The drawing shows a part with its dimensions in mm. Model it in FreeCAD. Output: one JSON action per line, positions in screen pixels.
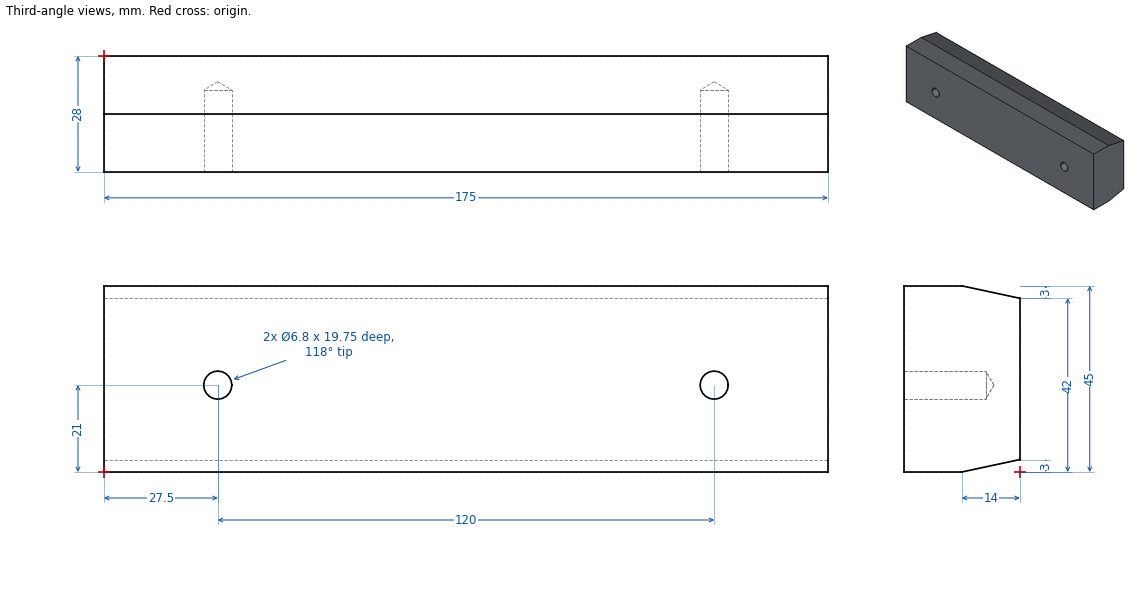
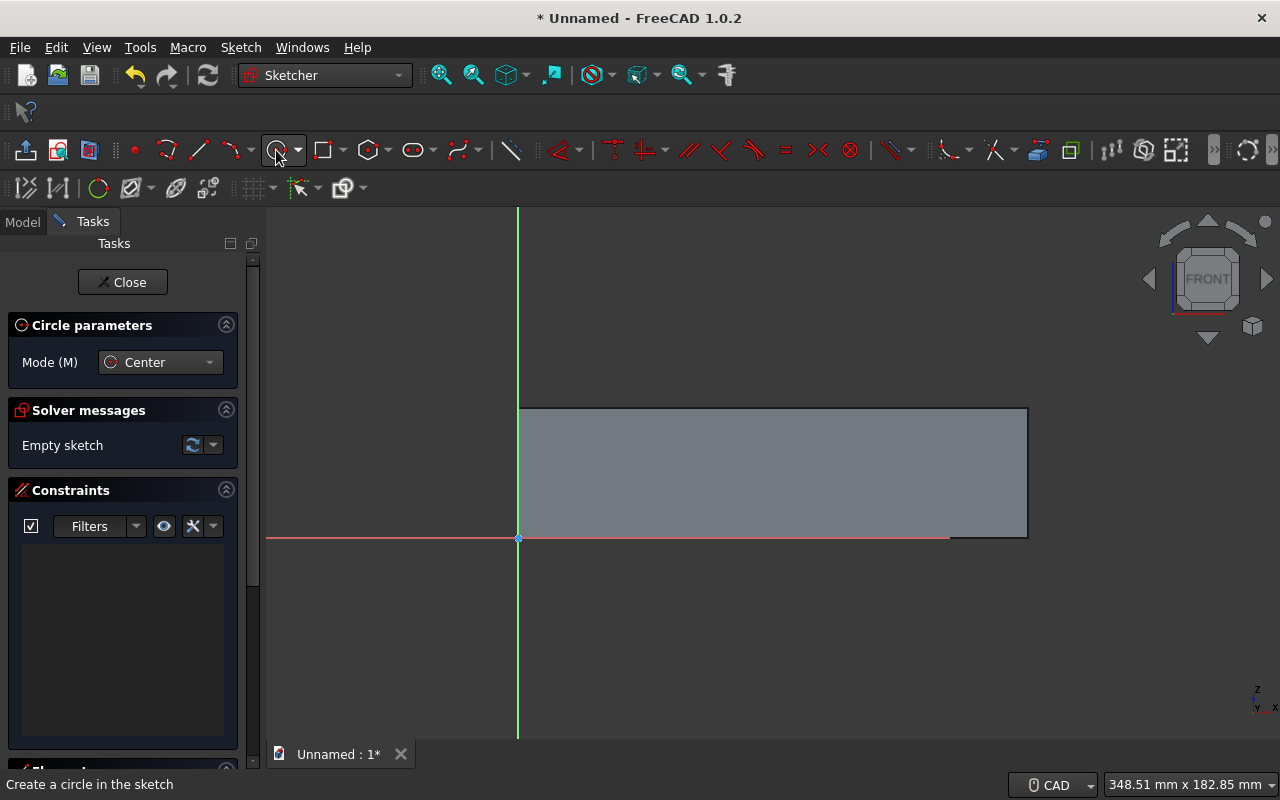
{"action": "scroll", "coordinate": [598, 477], "scroll_direction": "up", "scroll_amount": 5}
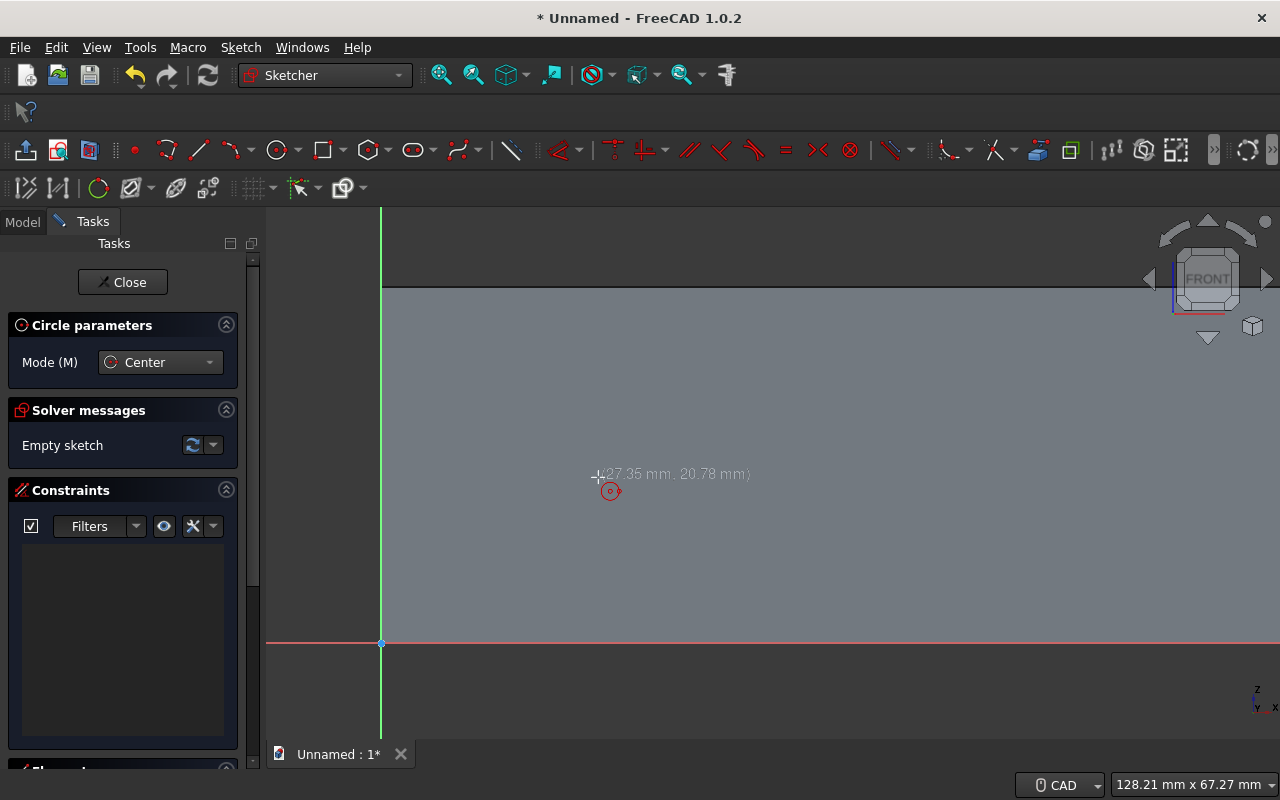
{"action": "left_click", "coordinate": [599, 477]}
{"action": "left_click", "coordinate": [618, 458]}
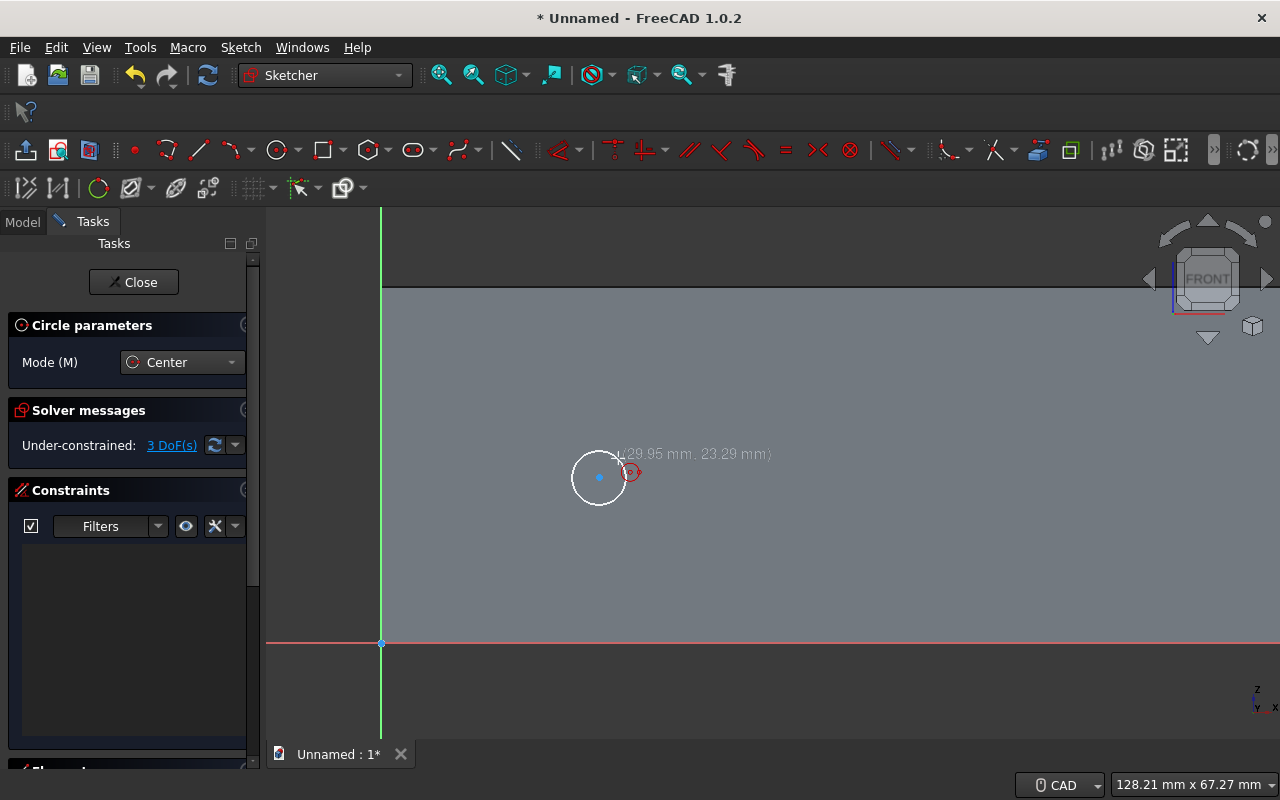
{"action": "scroll", "coordinate": [481, 413], "scroll_direction": "down", "scroll_amount": 4}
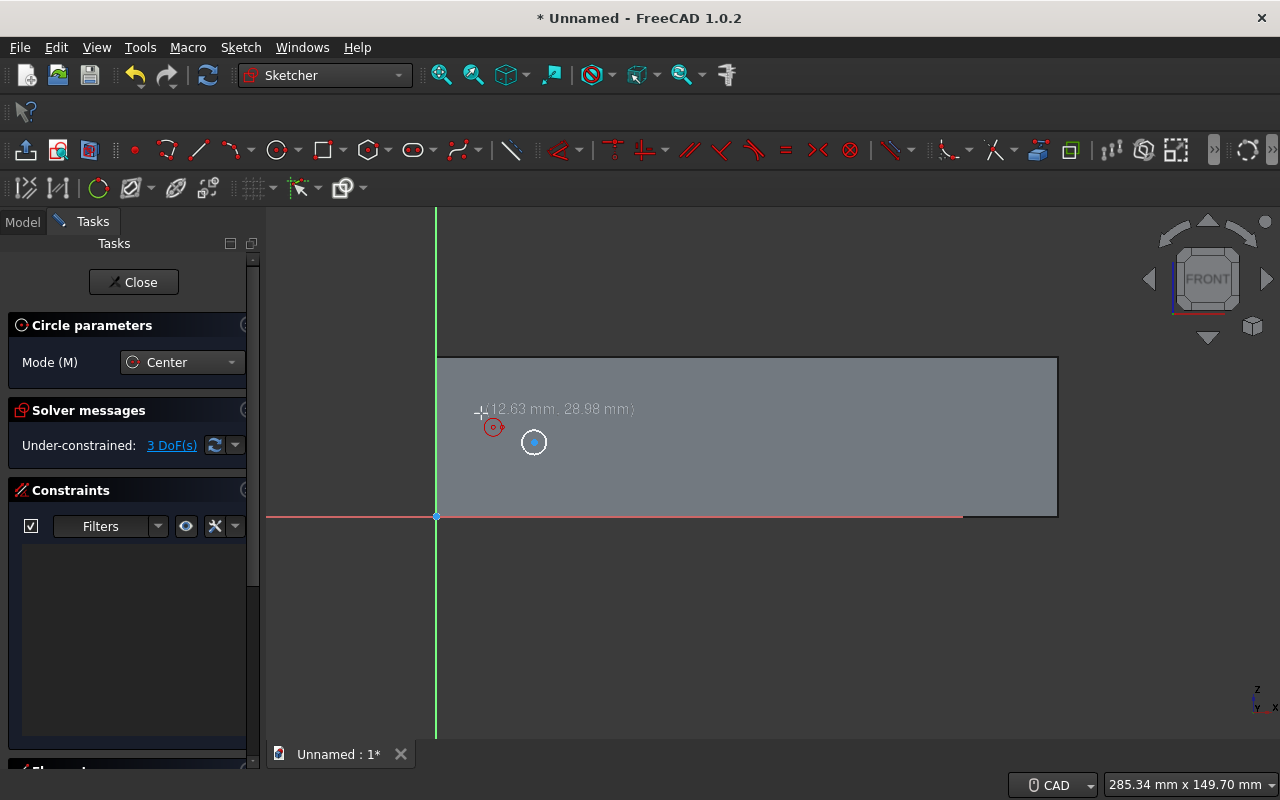
{"action": "scroll", "coordinate": [960, 442], "scroll_direction": "up", "scroll_amount": 4}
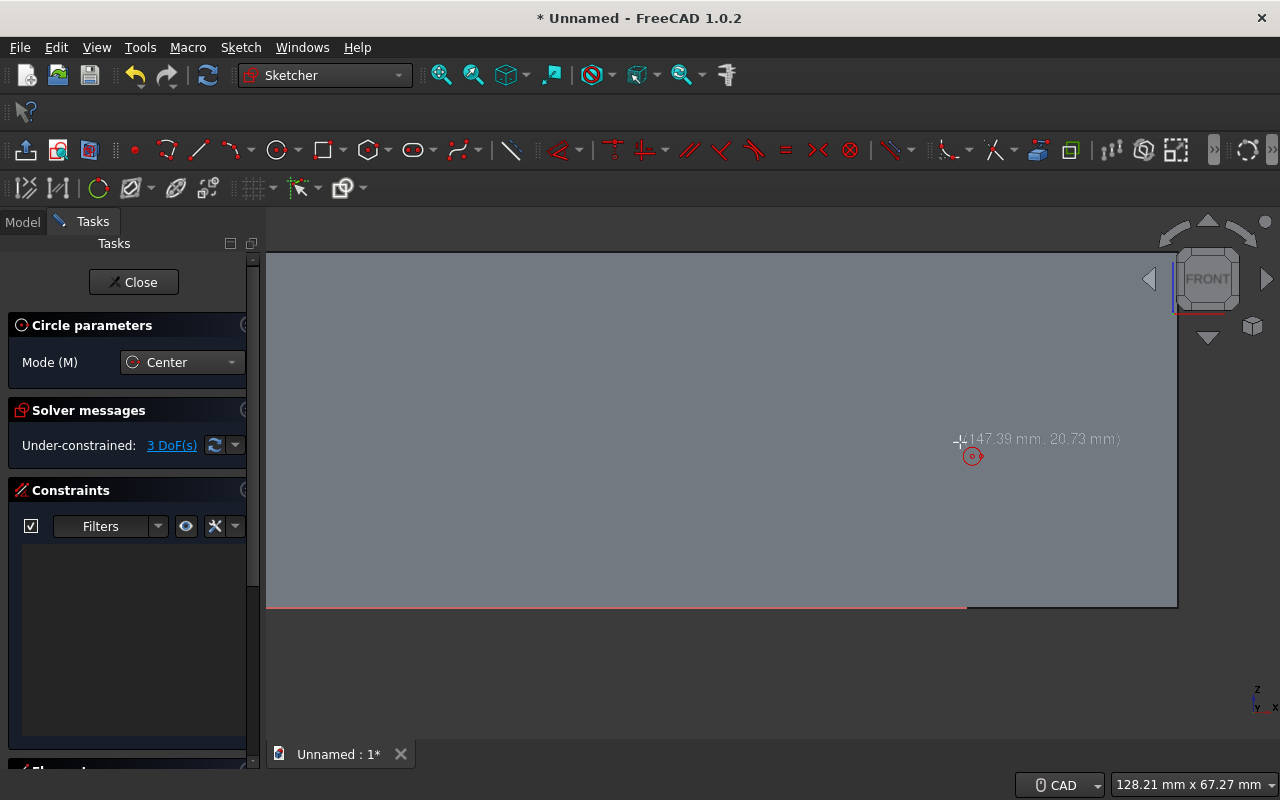
{"action": "left_click", "coordinate": [960, 442]}
{"action": "left_click", "coordinate": [979, 422]}
{"action": "key", "text": "Escape"}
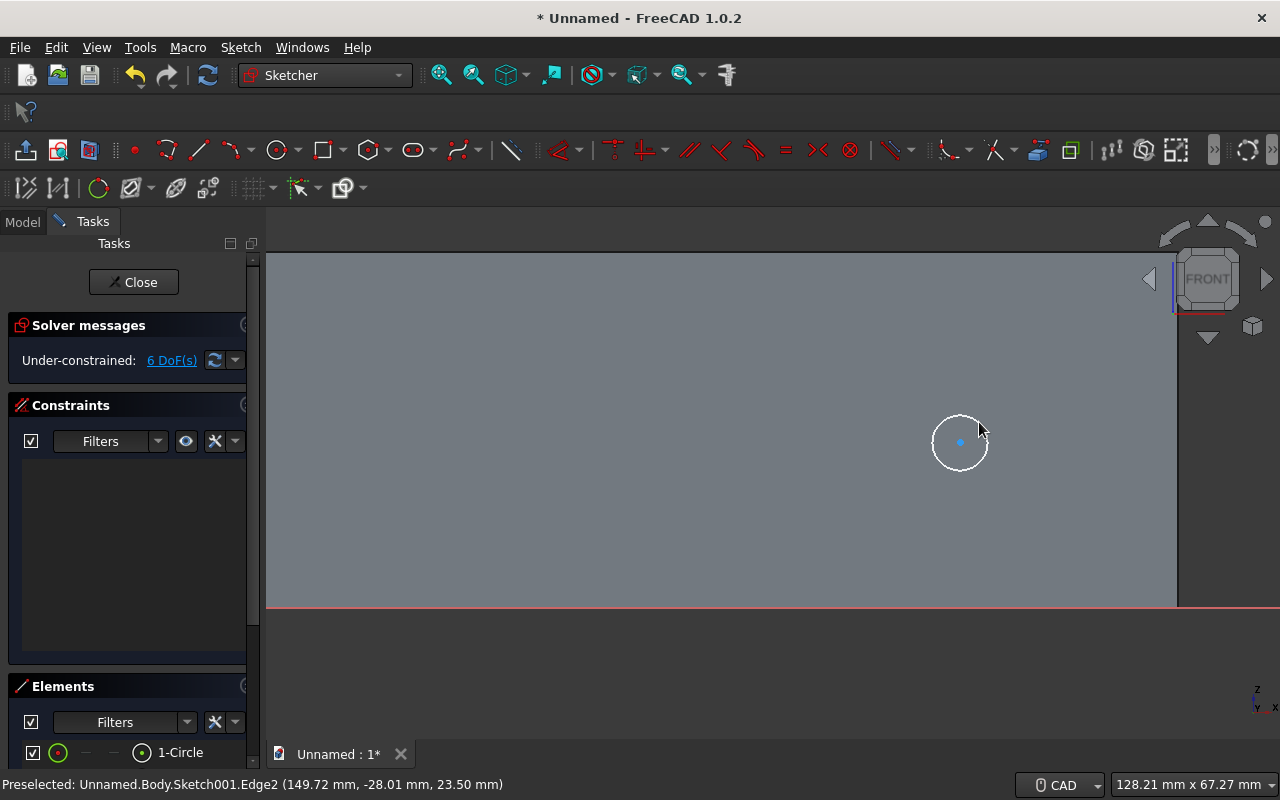
{"action": "scroll", "coordinate": [961, 442], "scroll_direction": "down", "scroll_amount": 4}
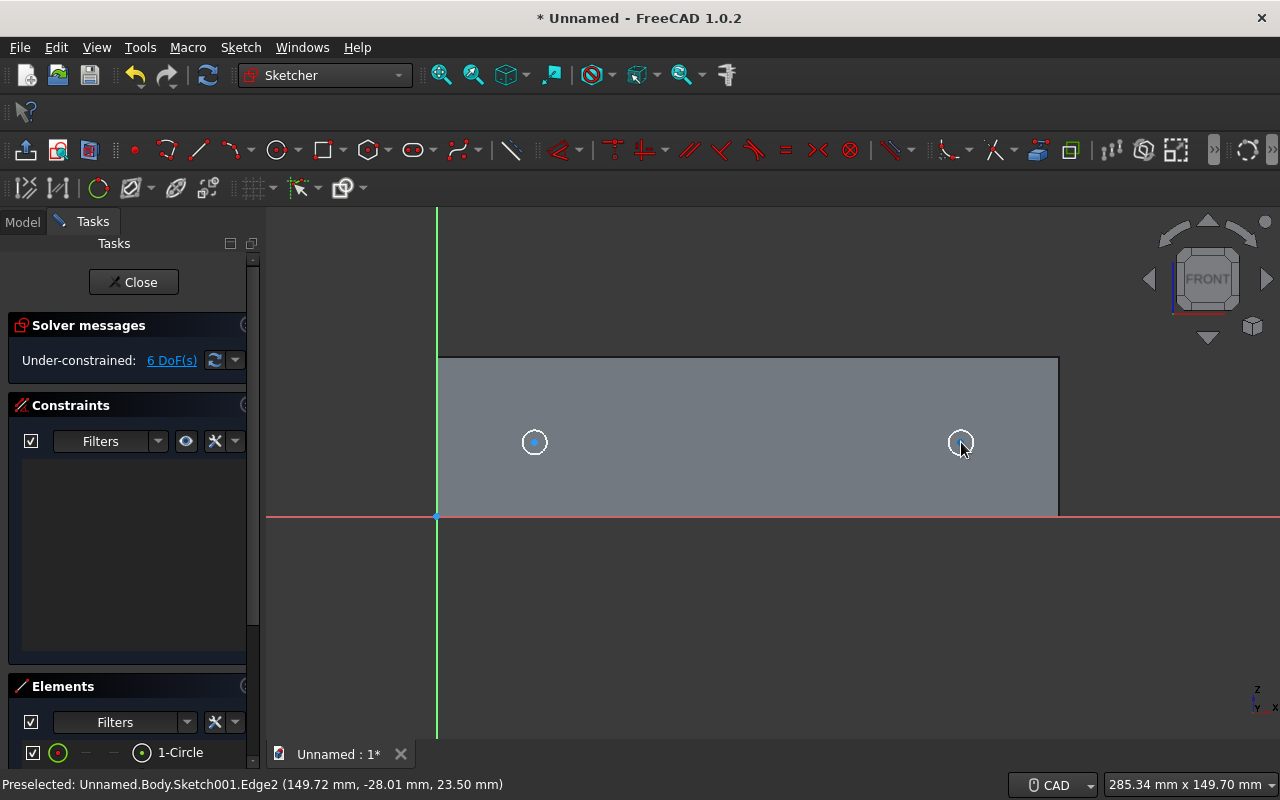
{"action": "left_click", "coordinate": [543, 434]}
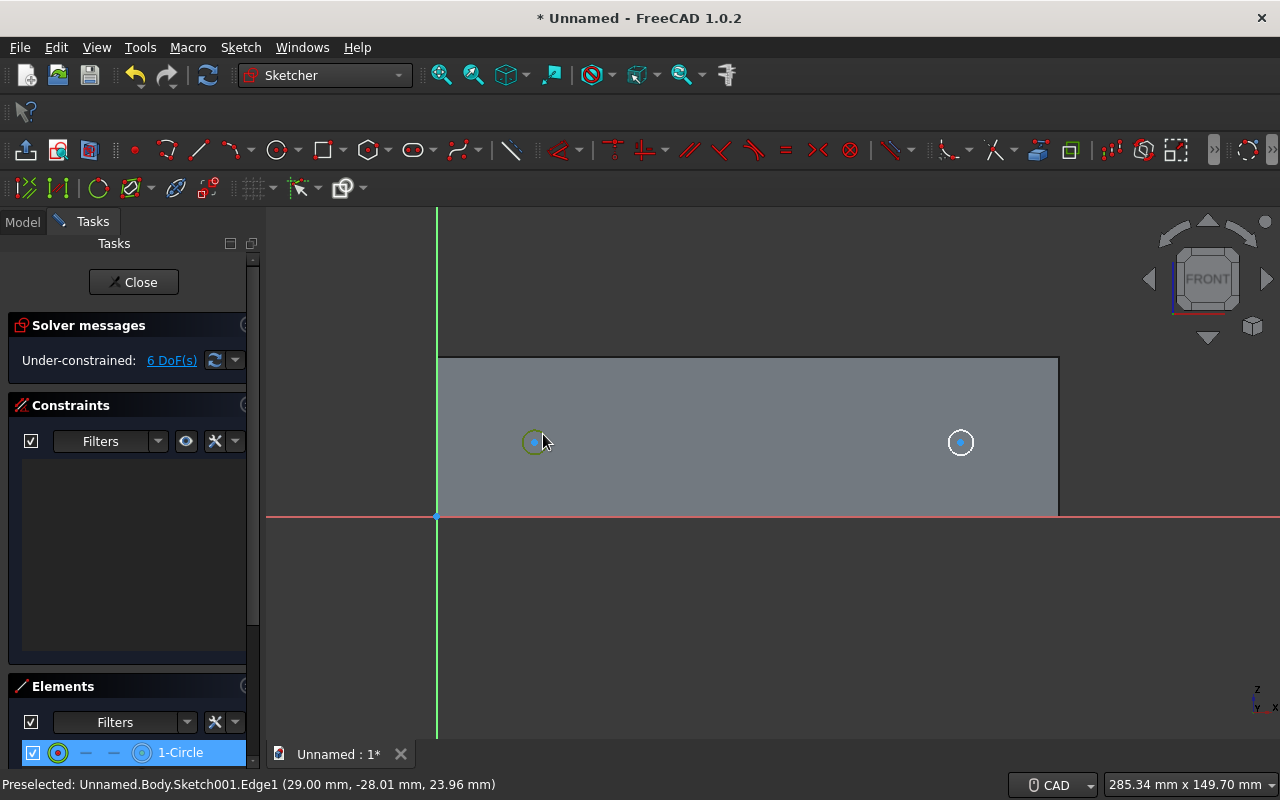
{"action": "left_click", "coordinate": [970, 434]}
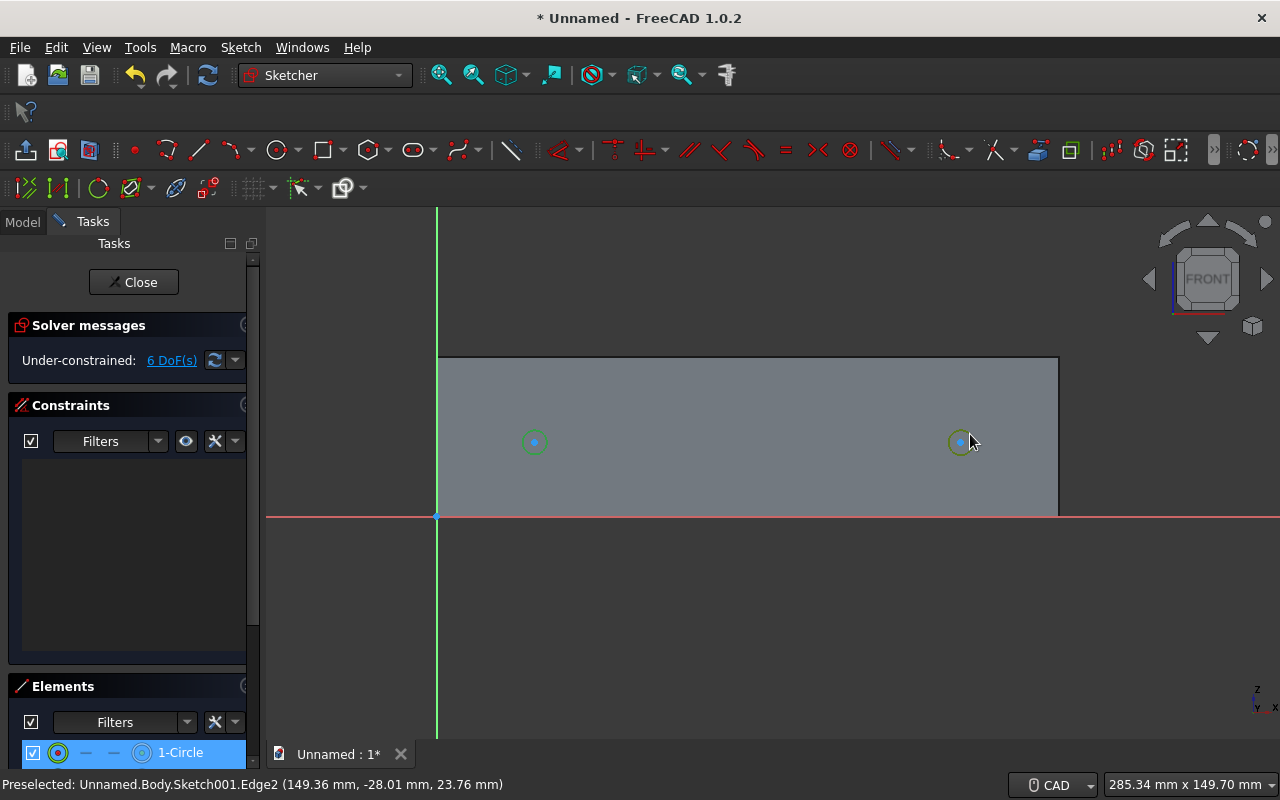
{"action": "key", "text": "e"}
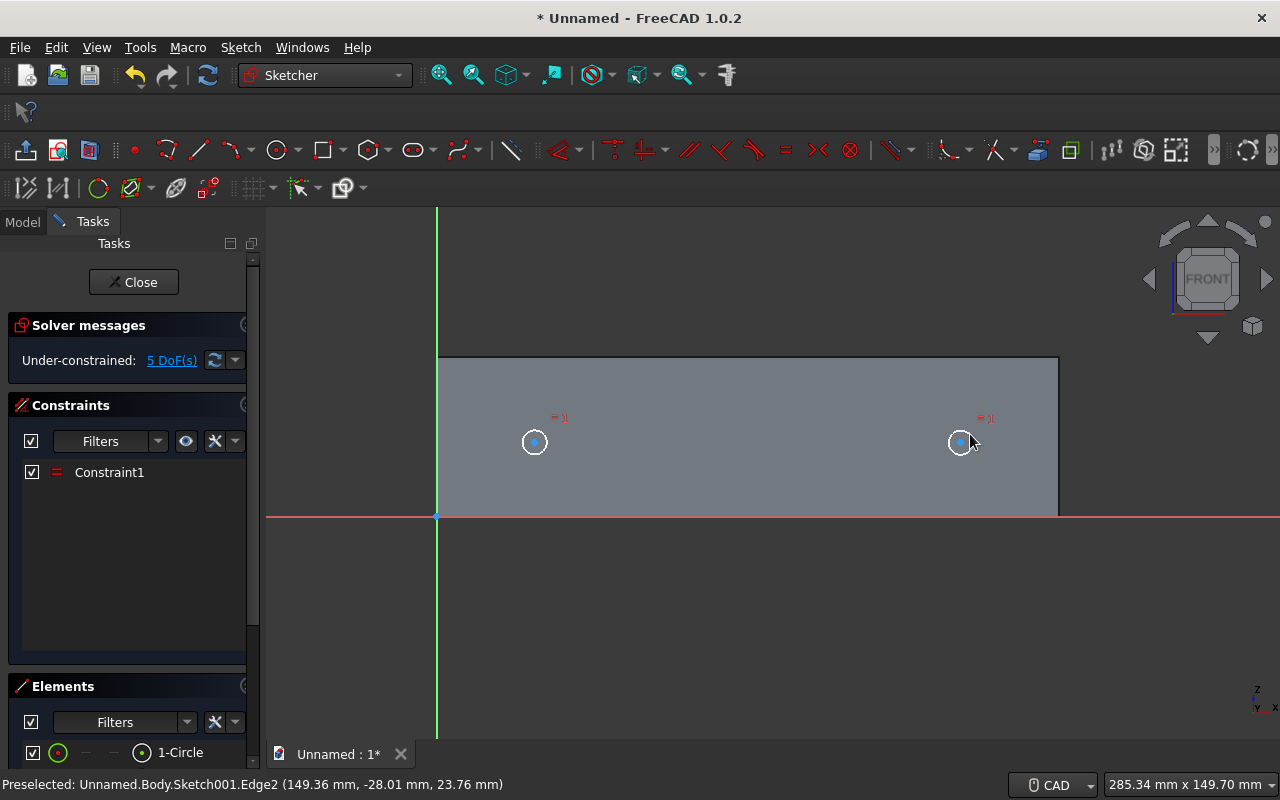
{"action": "key", "text": "d"}